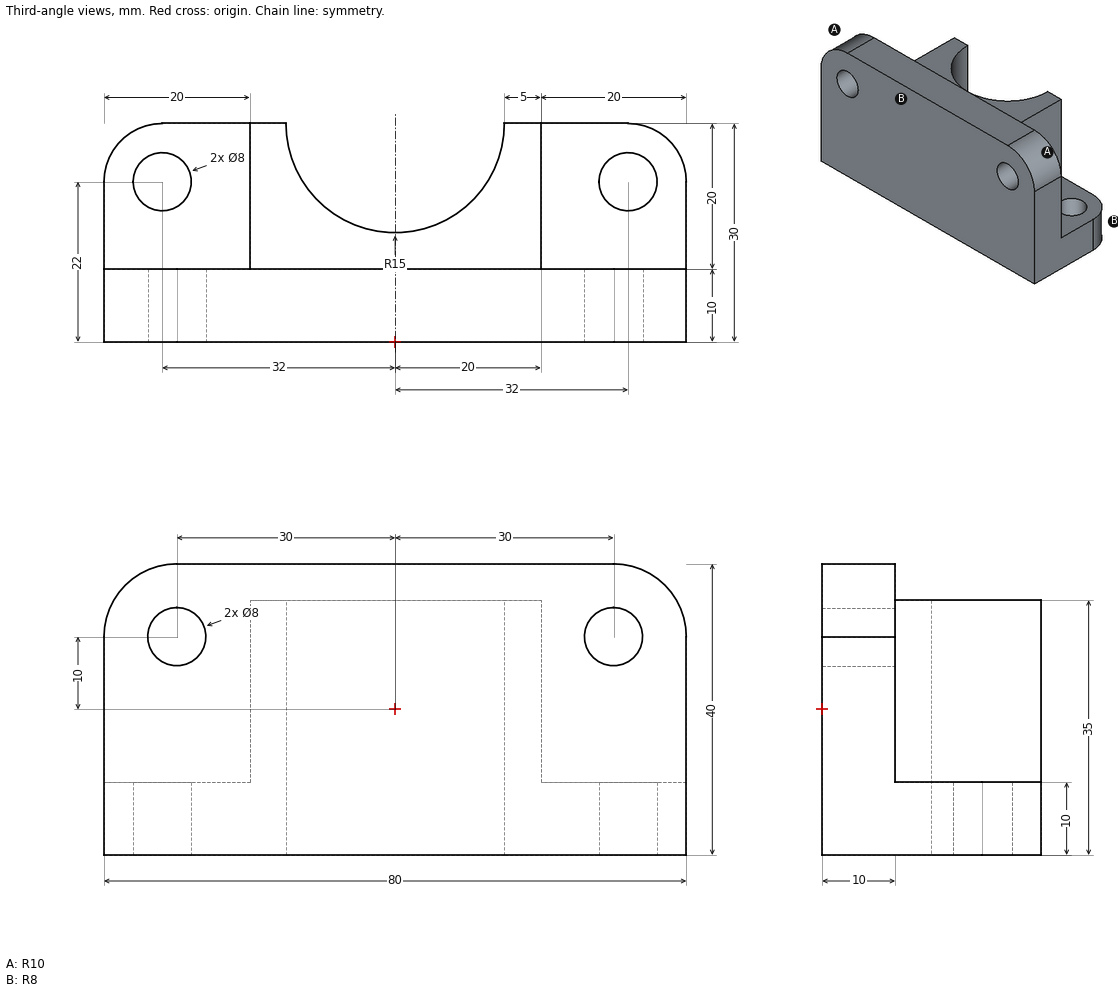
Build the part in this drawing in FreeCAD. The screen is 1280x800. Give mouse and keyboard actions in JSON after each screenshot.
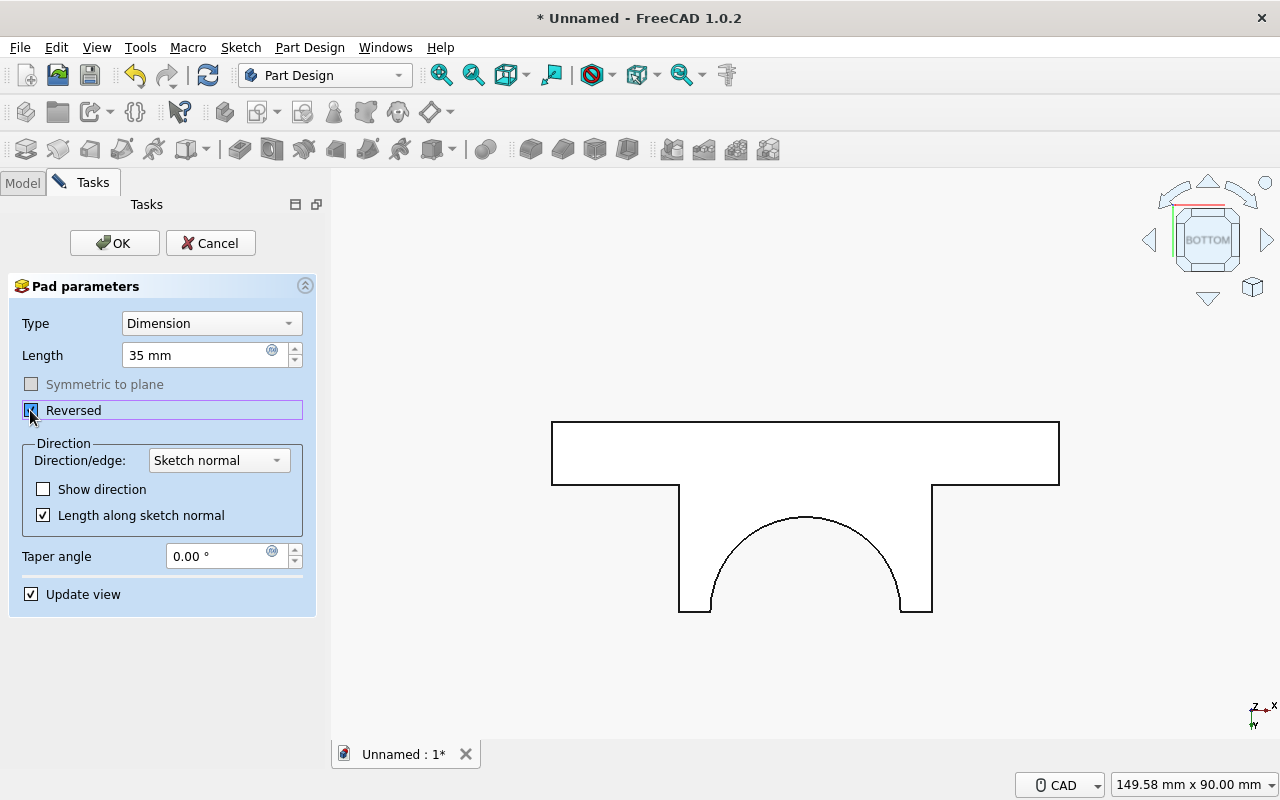
{"action": "left_click", "coordinate": [115, 243]}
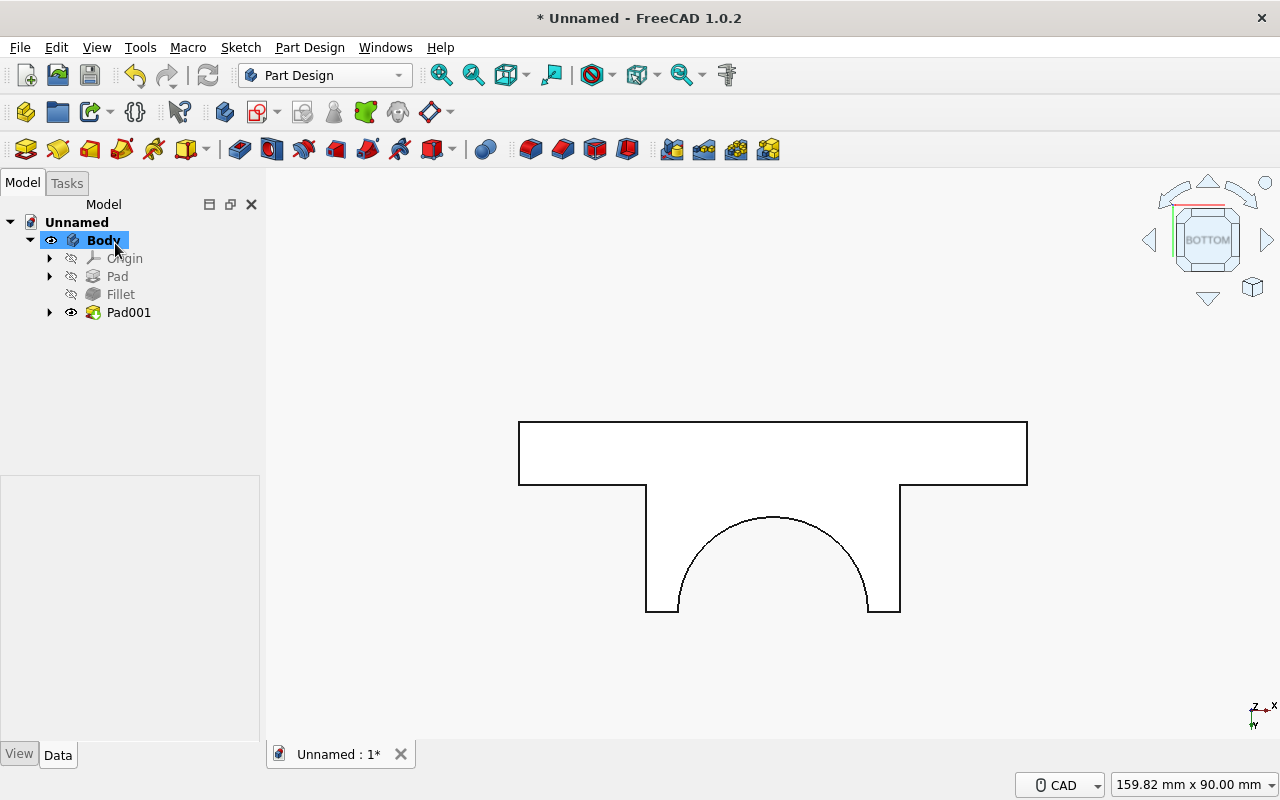
{"action": "left_click", "coordinate": [846, 489]}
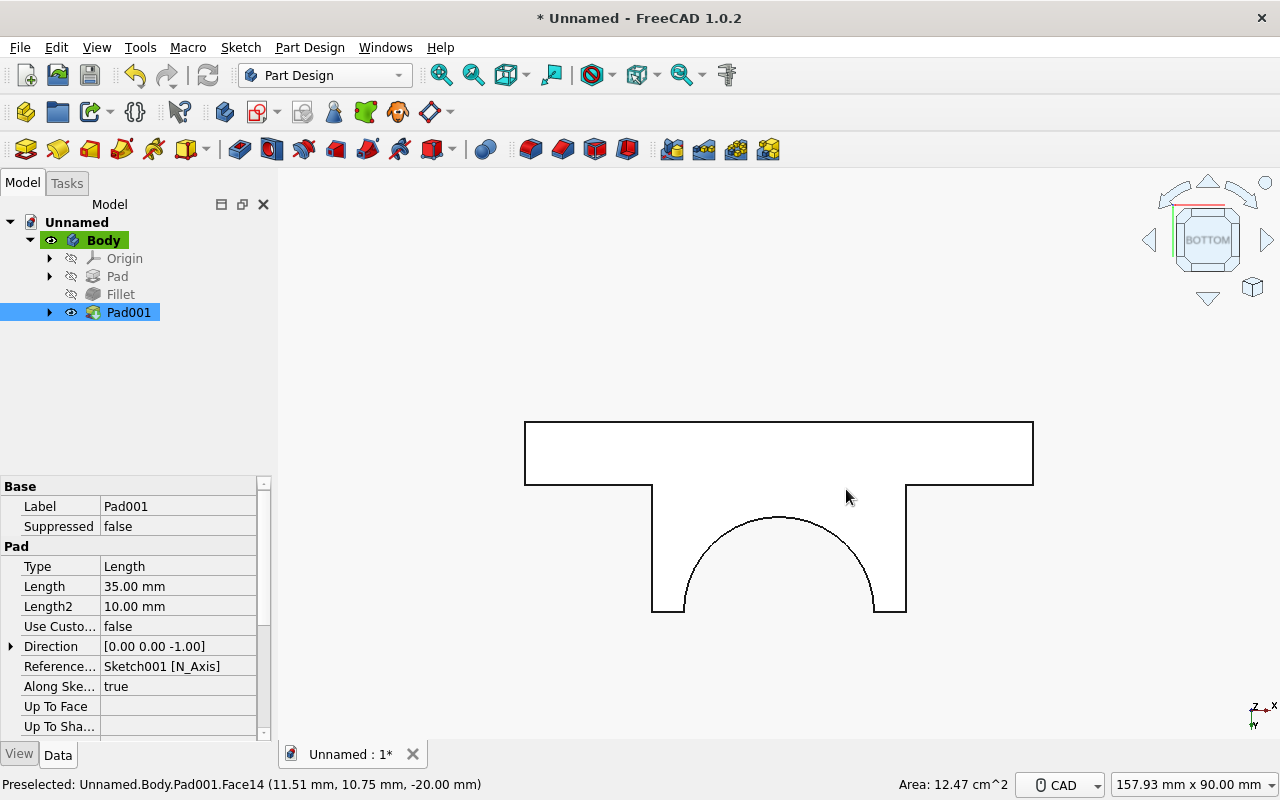
{"action": "left_click", "coordinate": [258, 112]}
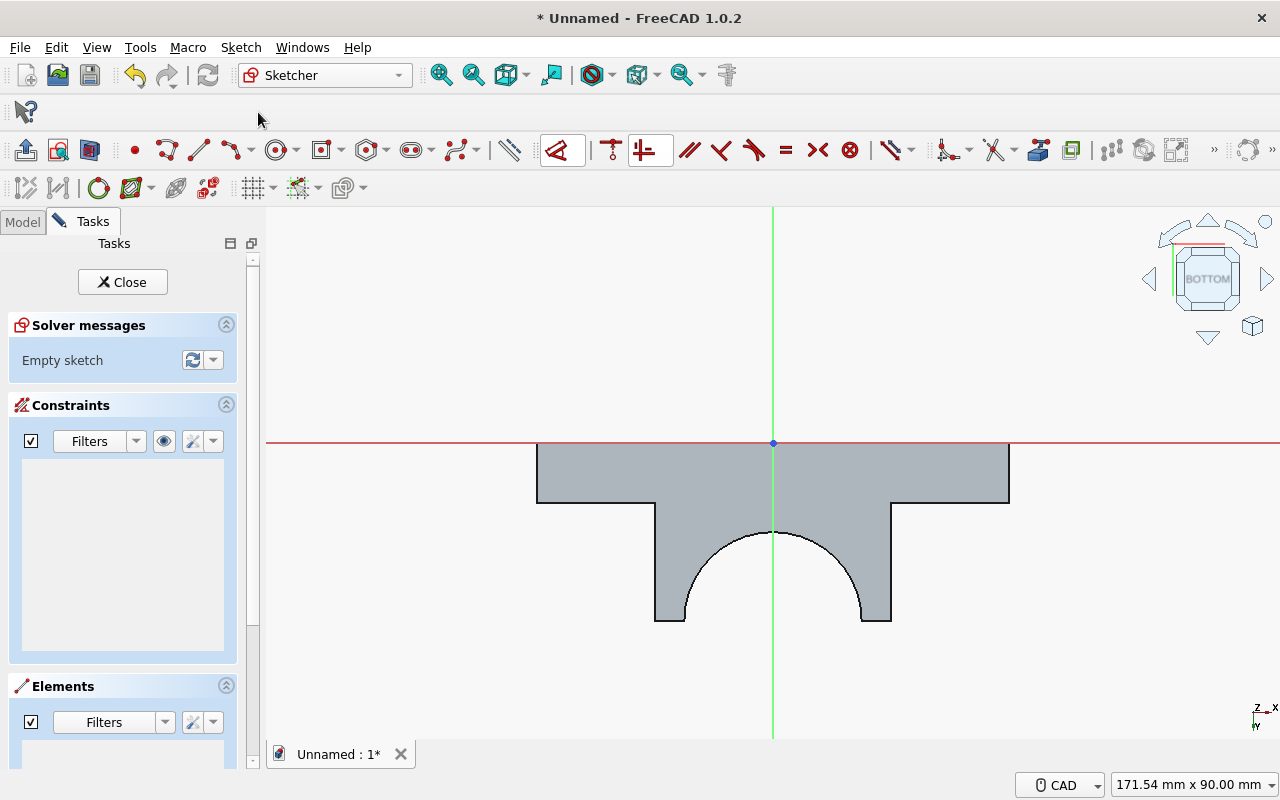
{"action": "left_click", "coordinate": [344, 150]}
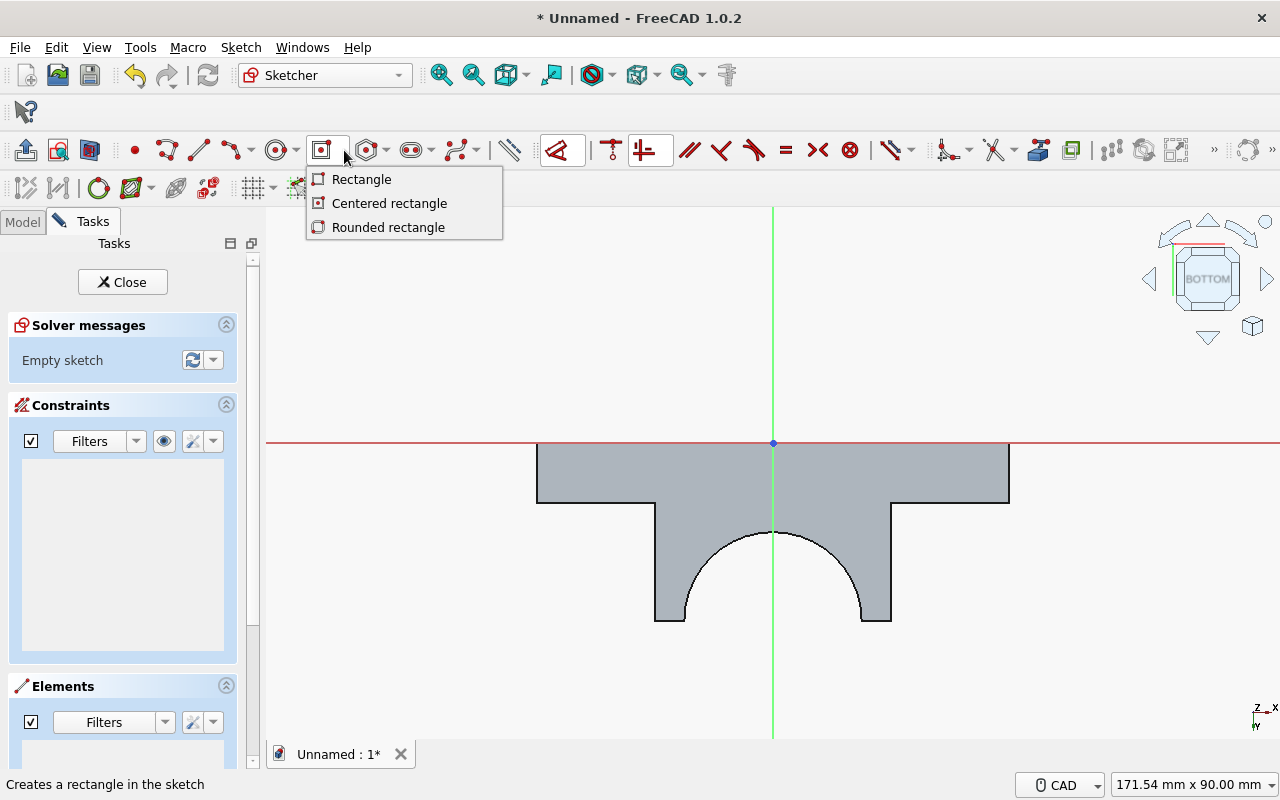
{"action": "left_click", "coordinate": [404, 179]}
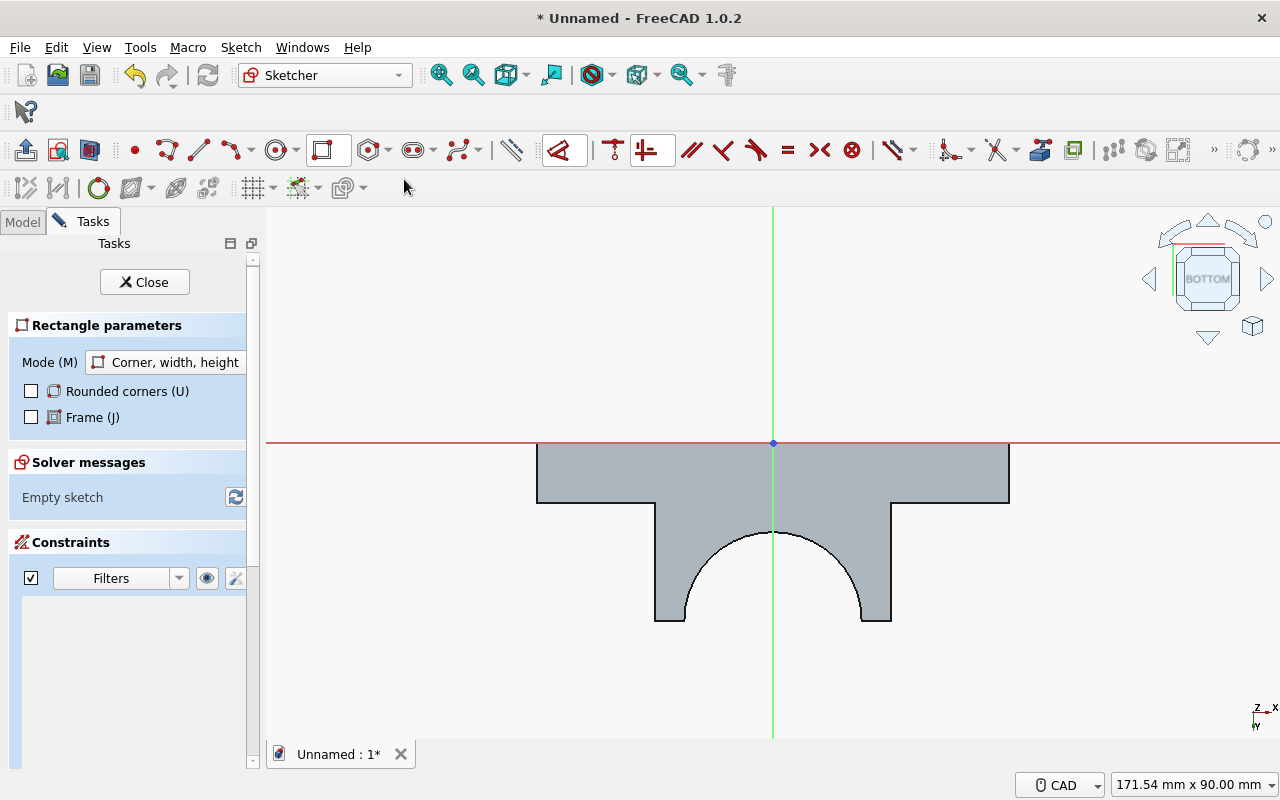
{"action": "left_click", "coordinate": [891, 503]}
{"action": "mouse_move", "coordinate": [1009, 621]}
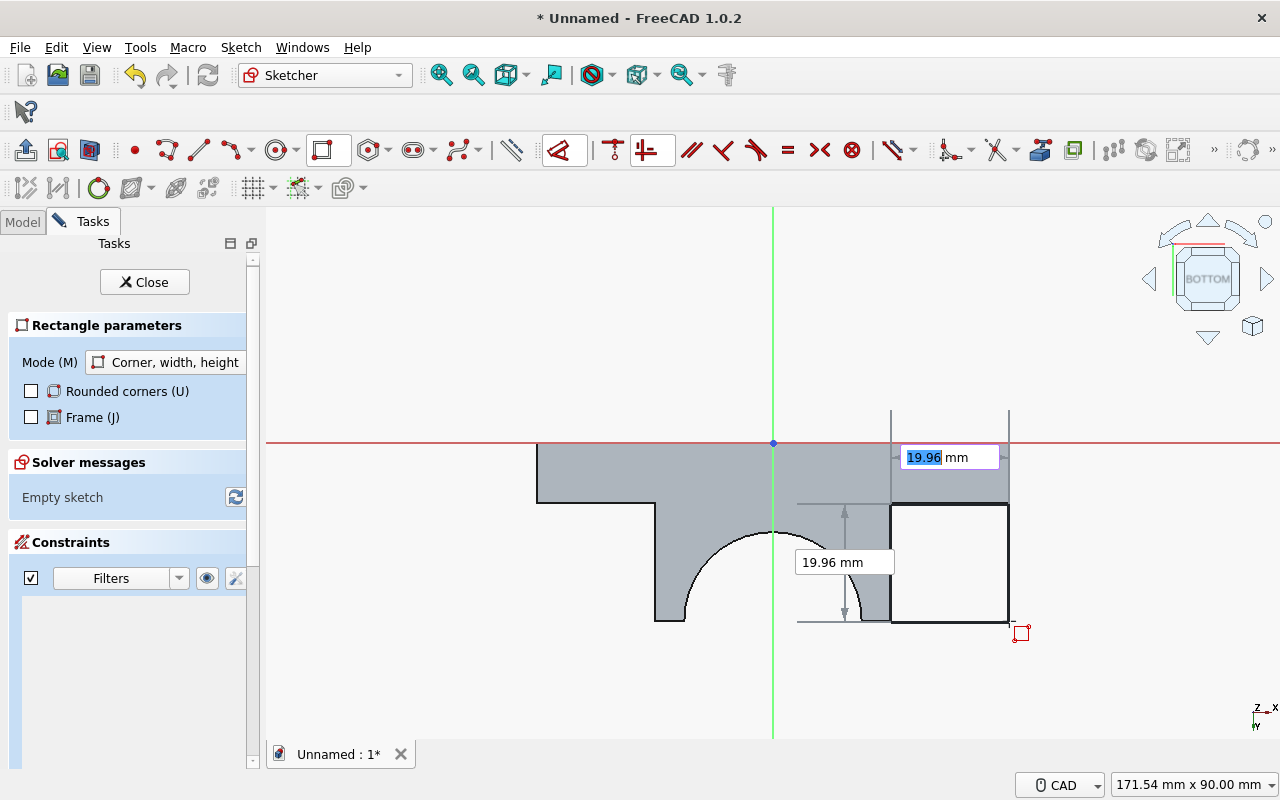
{"action": "type", "text": "20"}
{"action": "key", "text": "Tab"}
{"action": "type", "text": "20"}
{"action": "key", "text": "Return"}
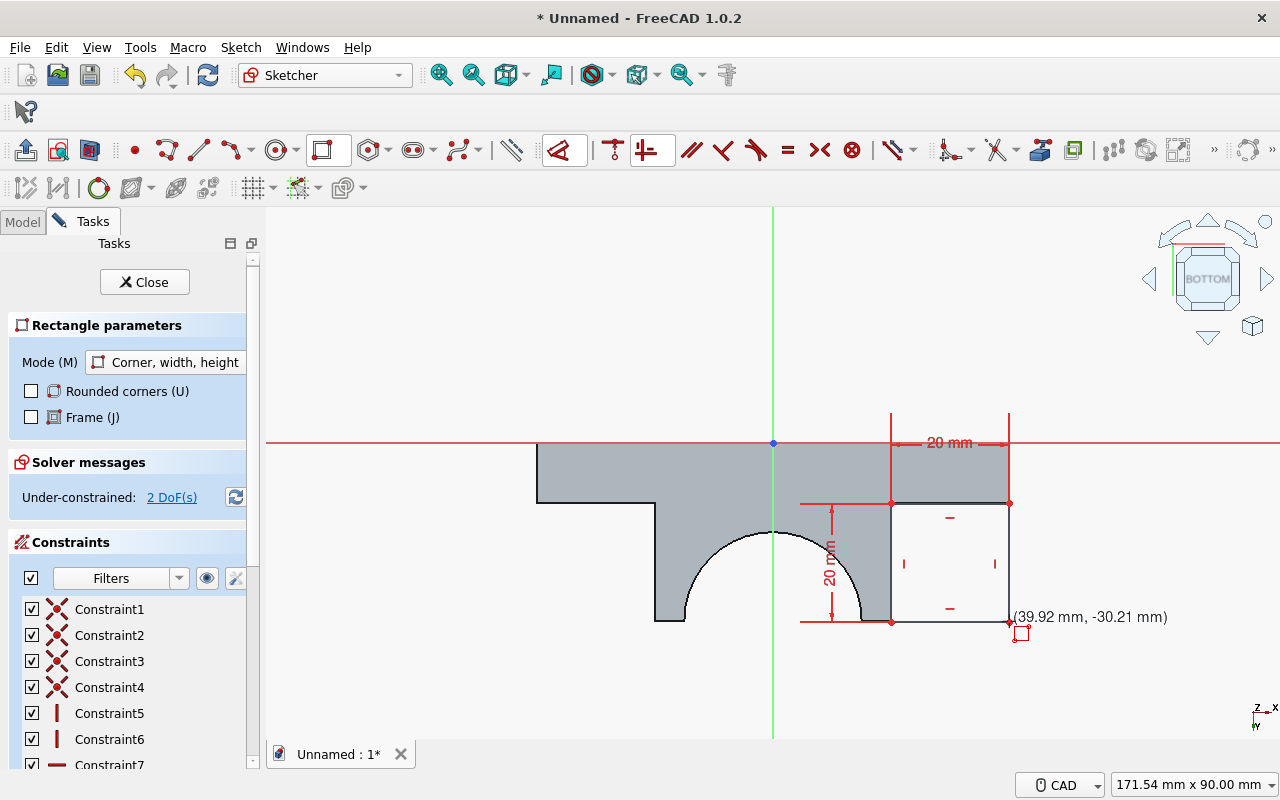
{"action": "left_click", "coordinate": [537, 503]}
{"action": "mouse_move", "coordinate": [655, 621]}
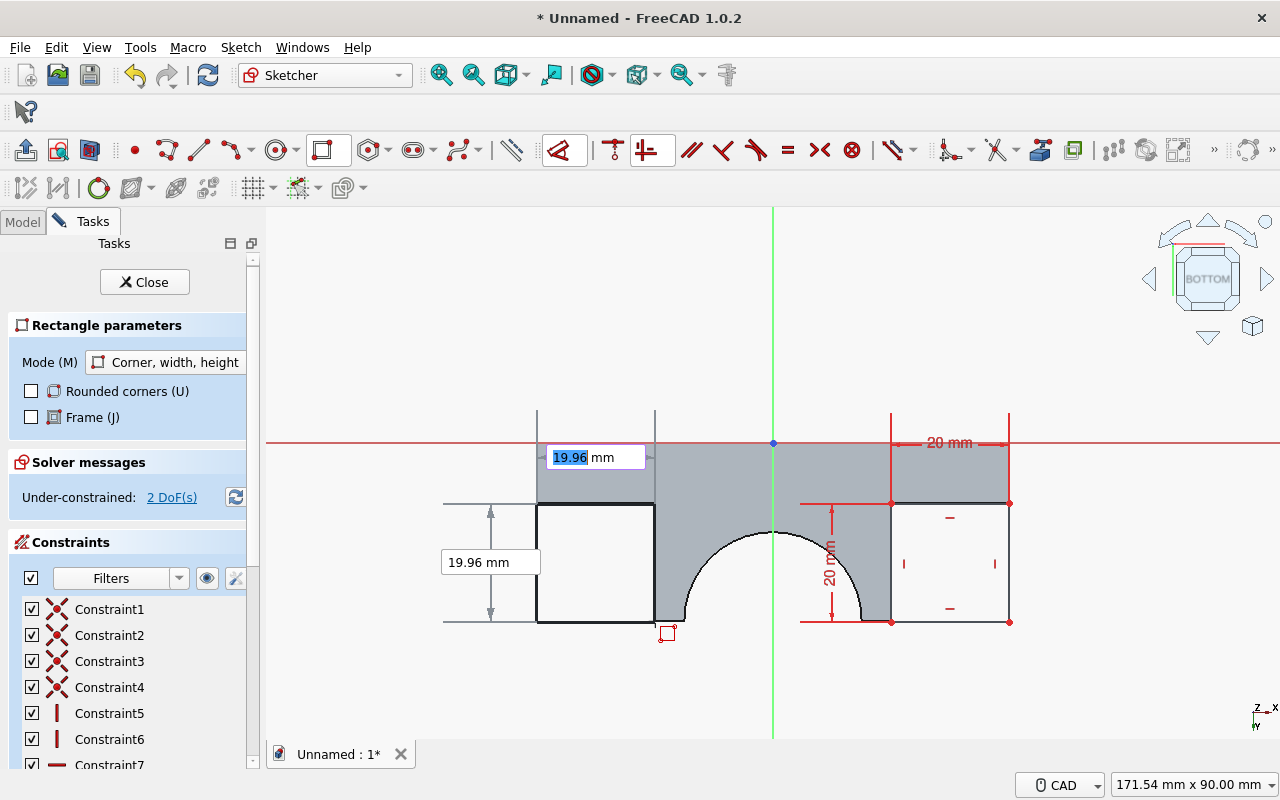
{"action": "type", "text": "20"}
{"action": "key", "text": "Tab"}
{"action": "type", "text": "20"}
{"action": "key", "text": "Return"}
{"action": "key", "text": "Escape"}